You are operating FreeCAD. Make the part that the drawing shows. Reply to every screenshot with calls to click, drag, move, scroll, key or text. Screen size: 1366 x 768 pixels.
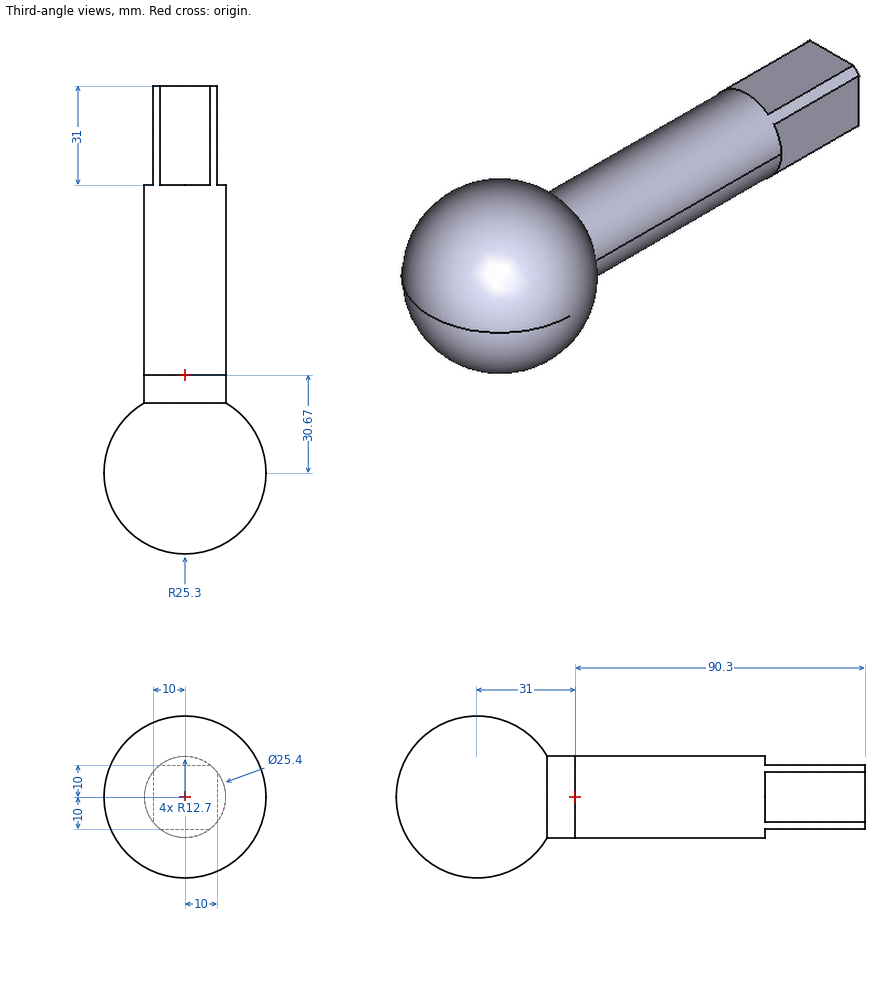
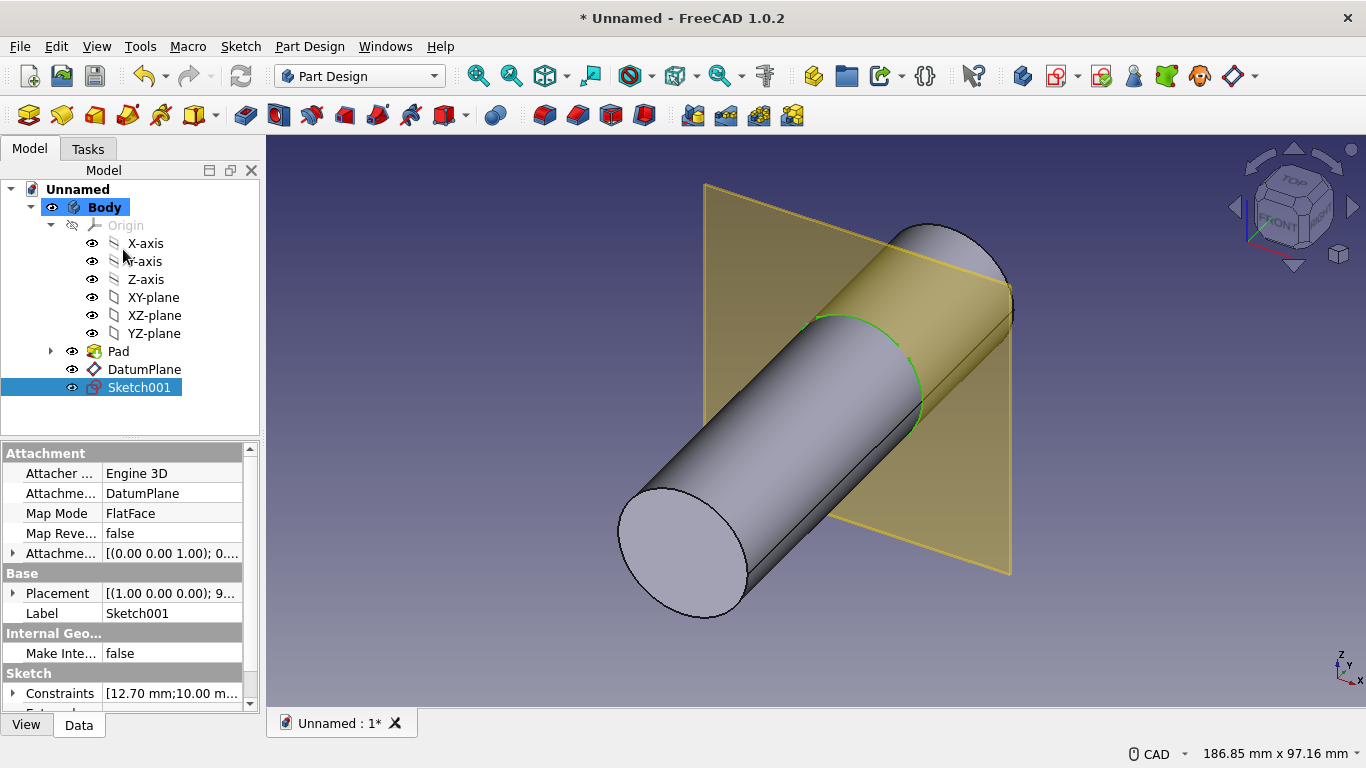
click(246, 116)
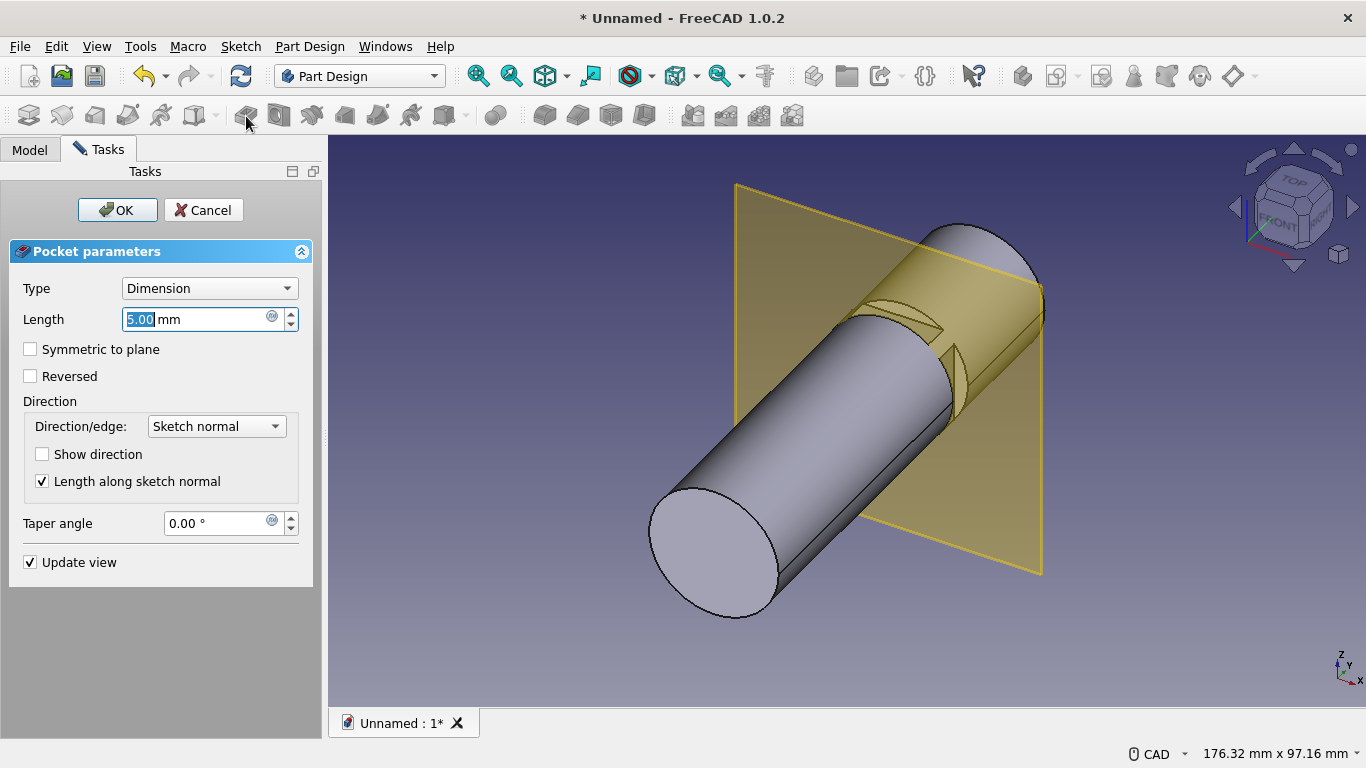
text(31)
key(Tab)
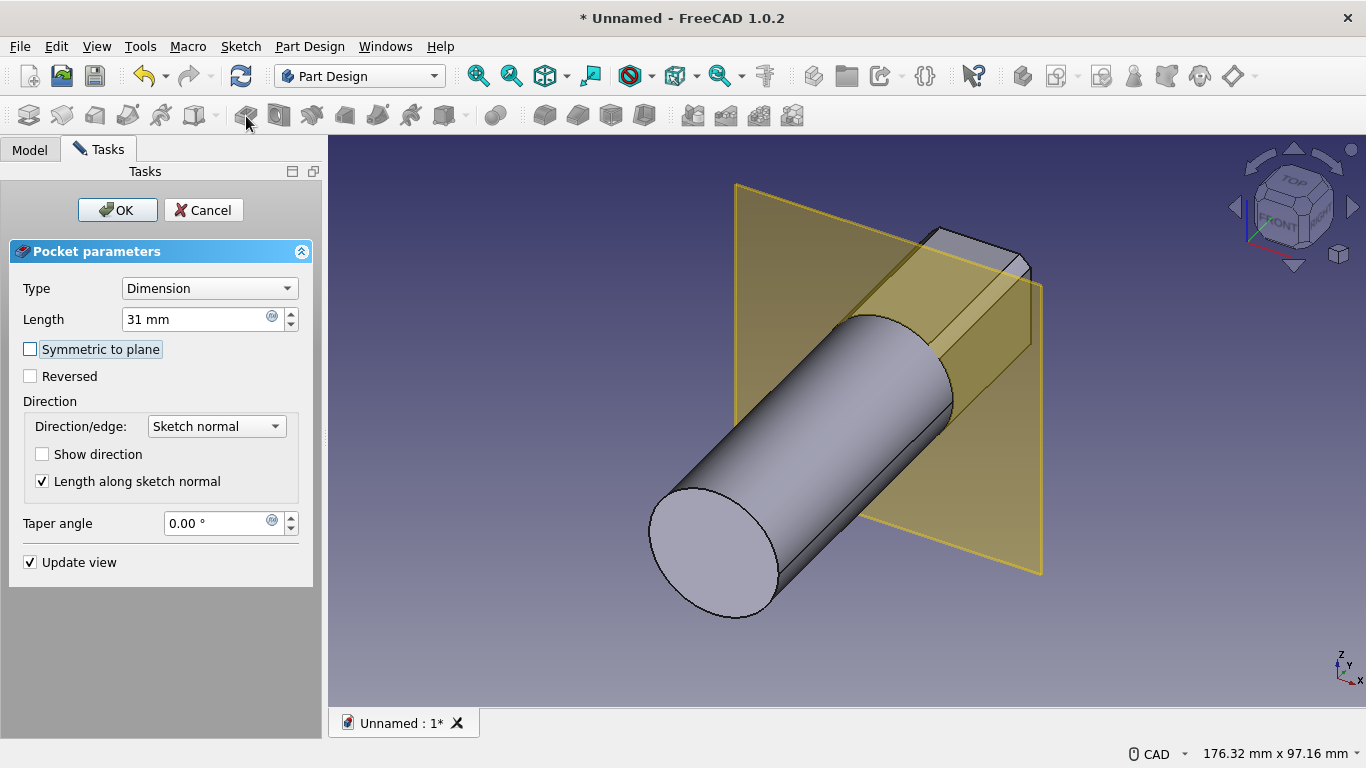
click(118, 210)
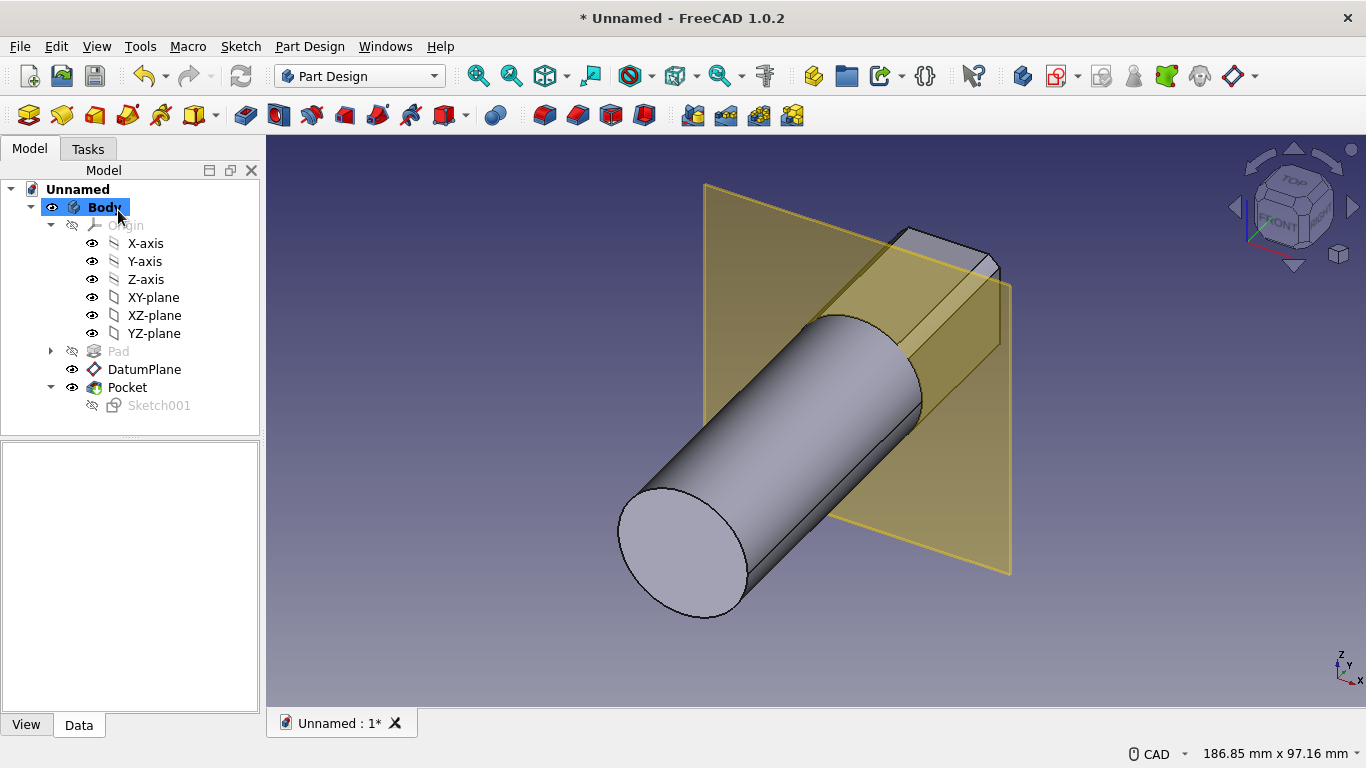
click(117, 369)
key(space)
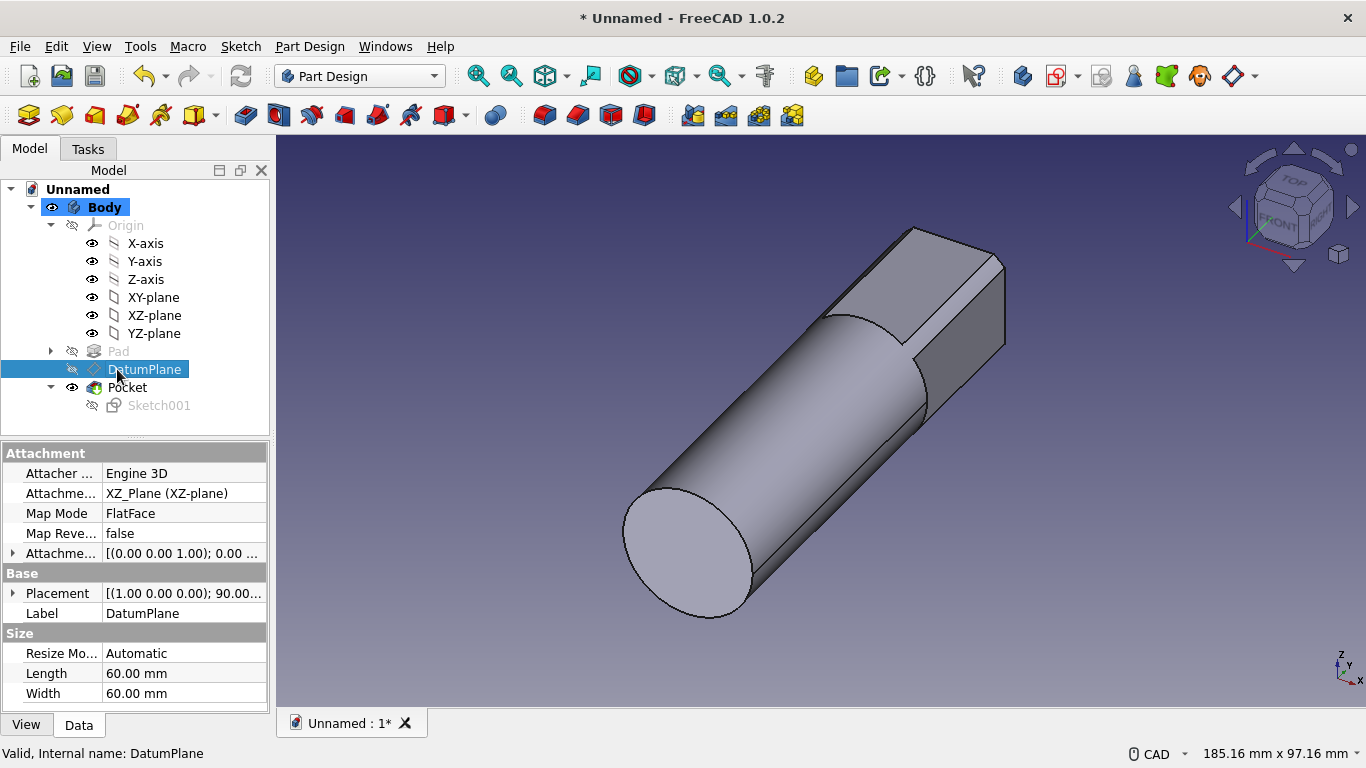
click(137, 315)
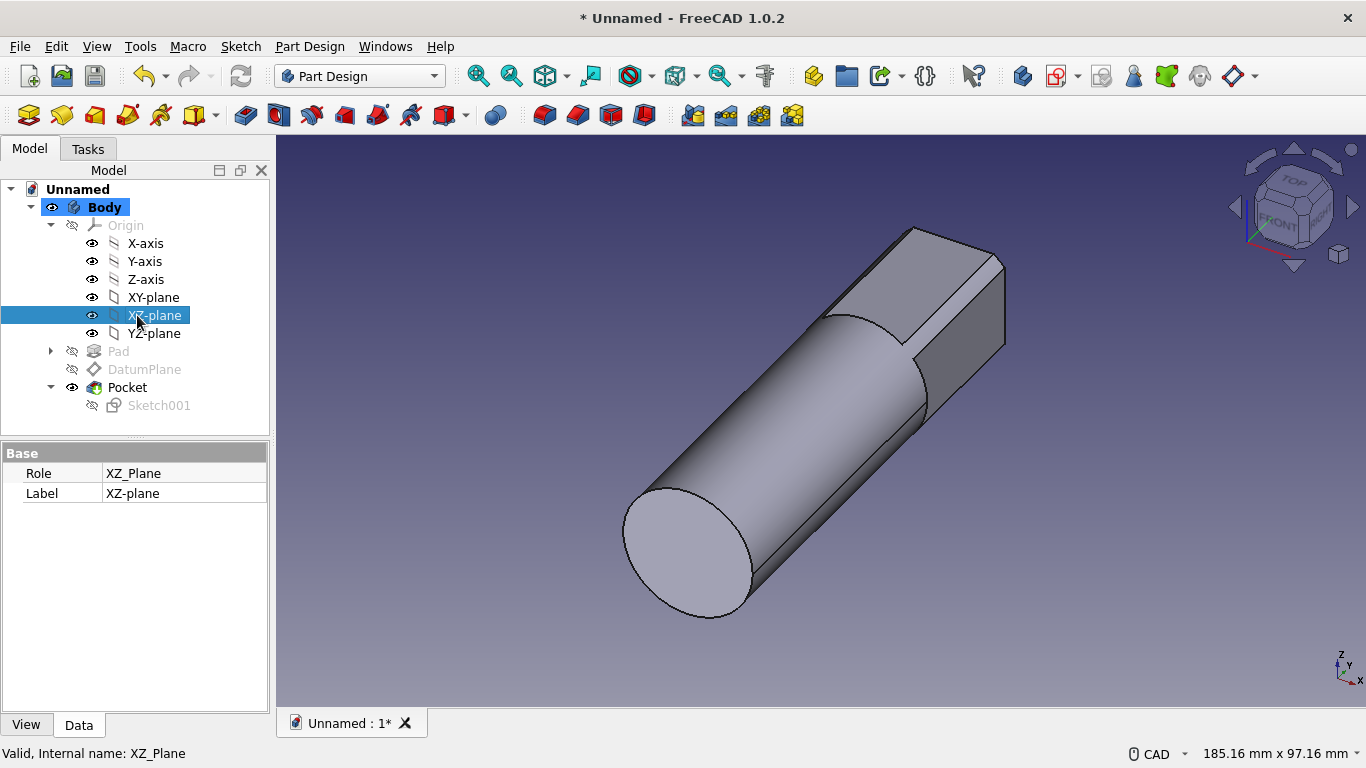
click(1232, 76)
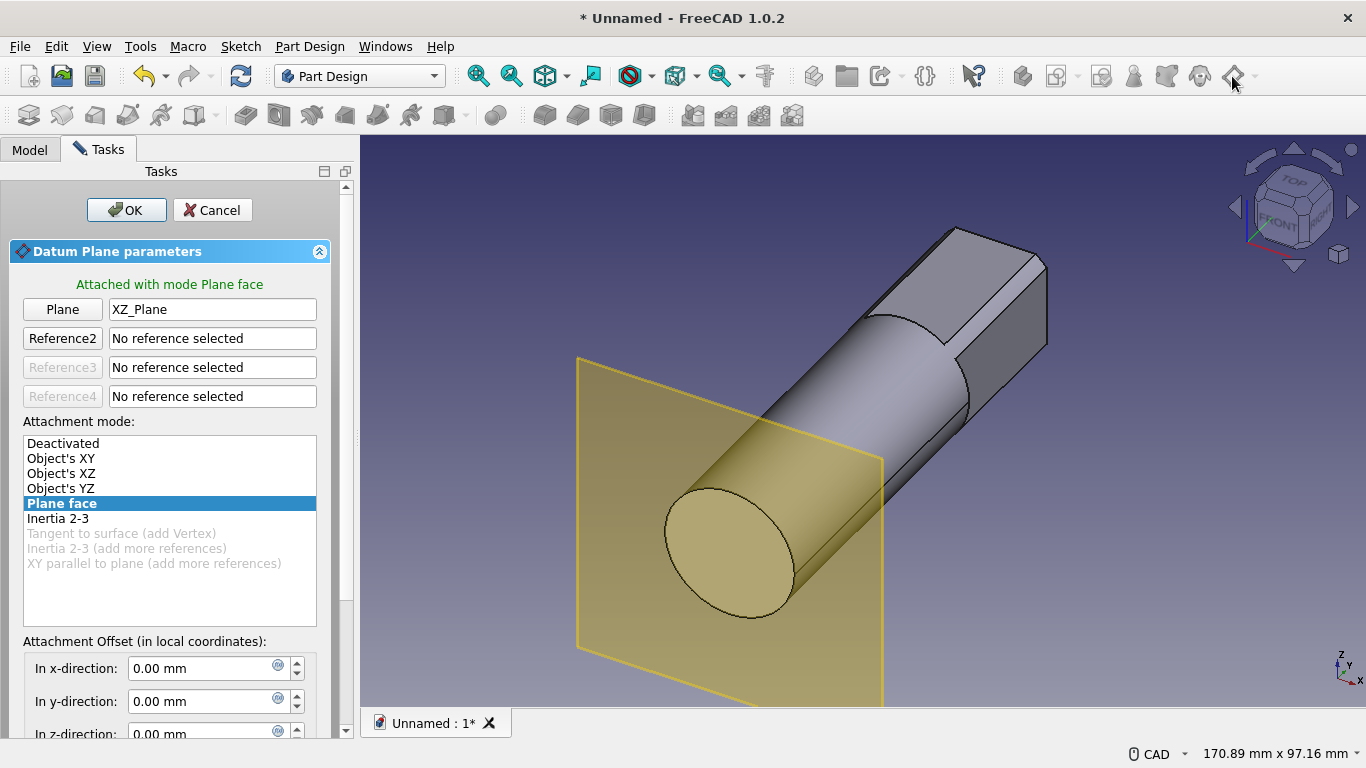
scroll(346, 460, down, 2)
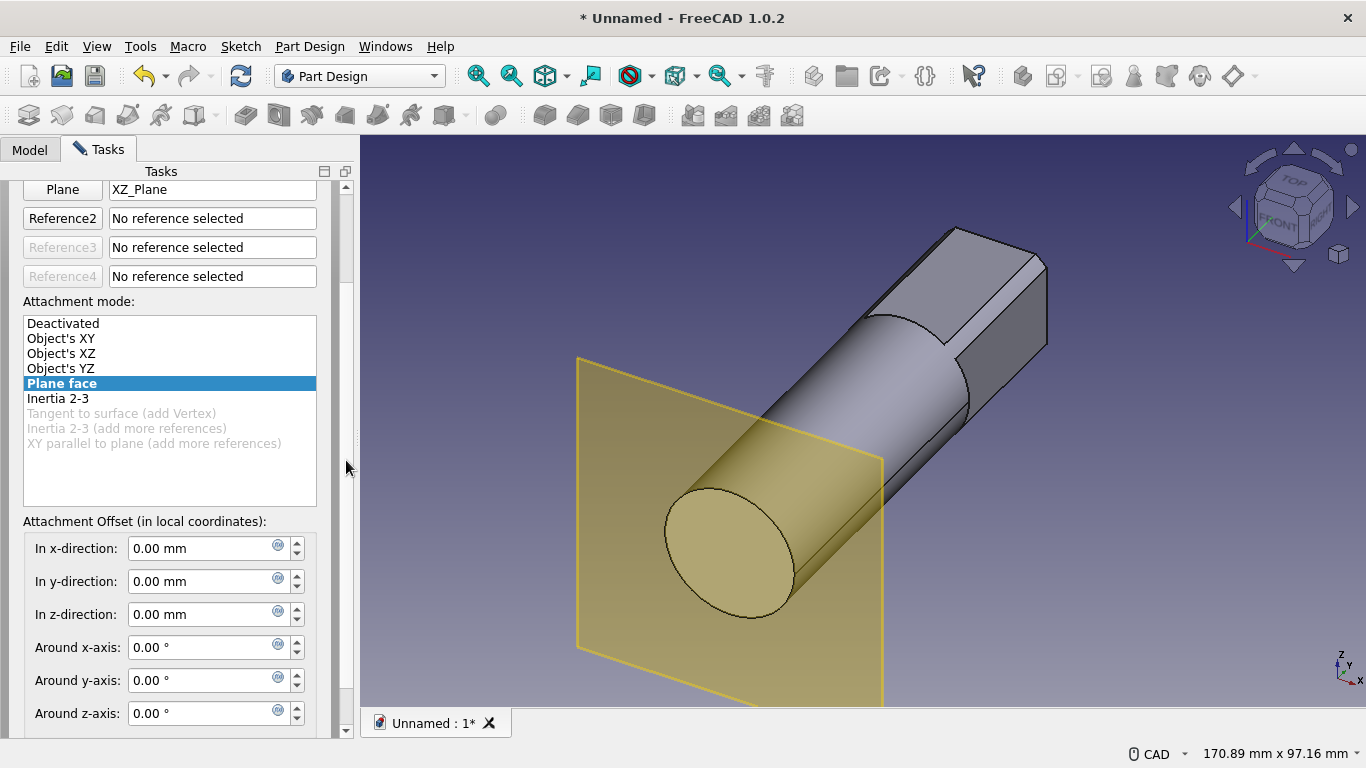
triple_click(210, 614)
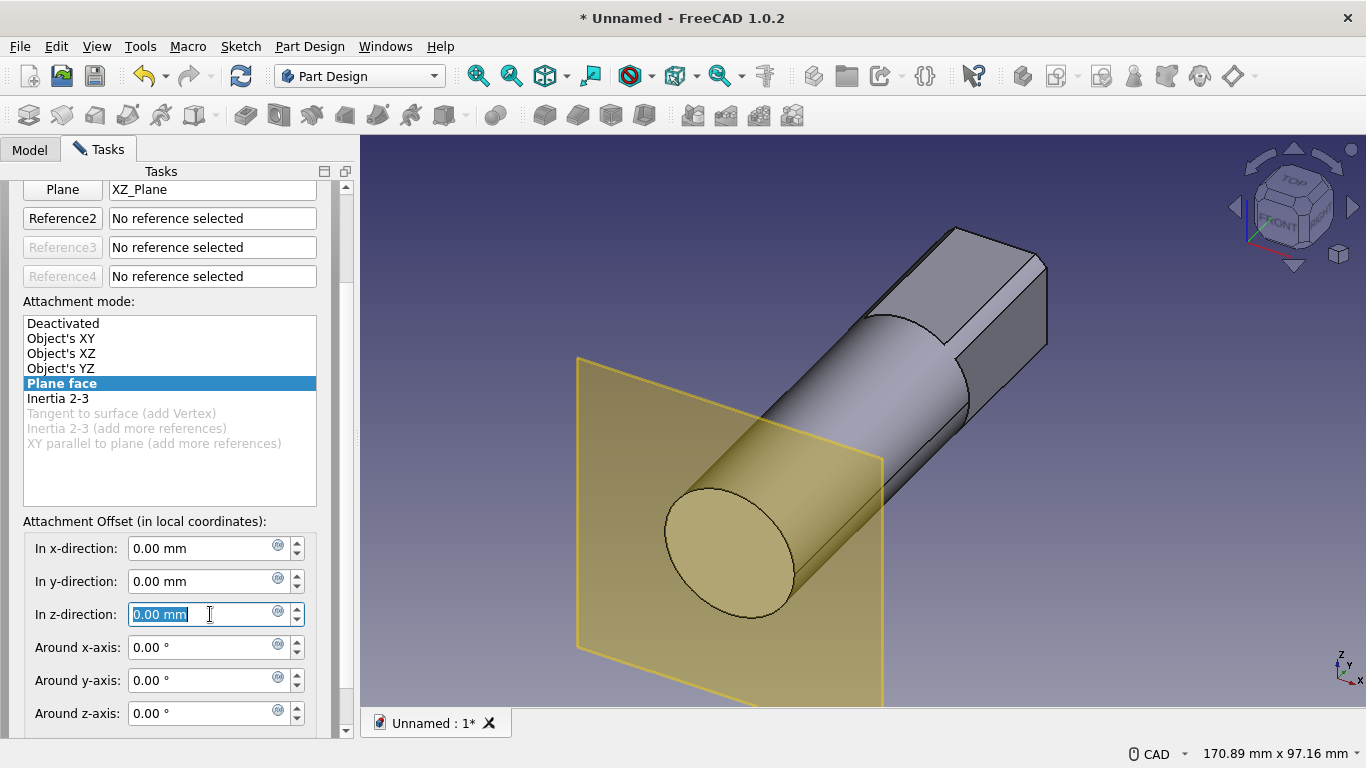
text(31)
key(Tab)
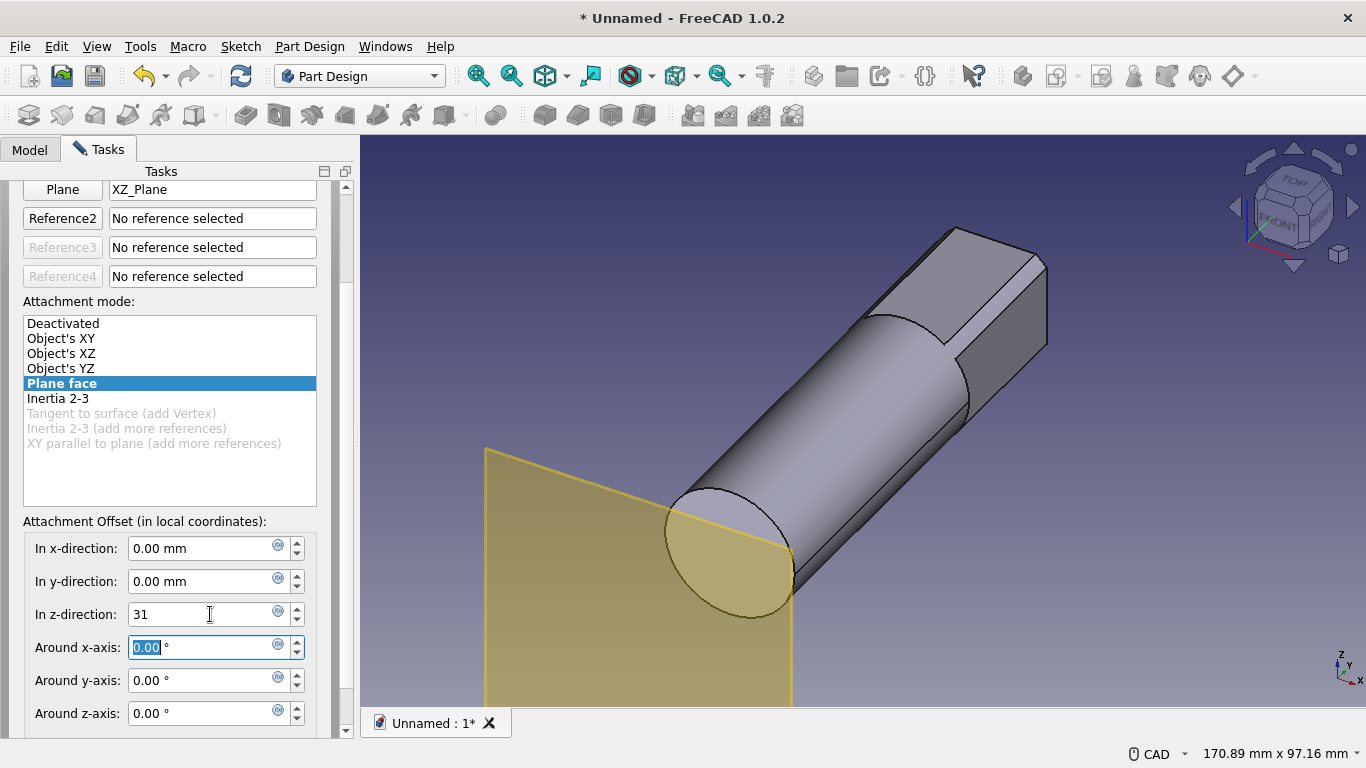
scroll(346, 460, up, 3)